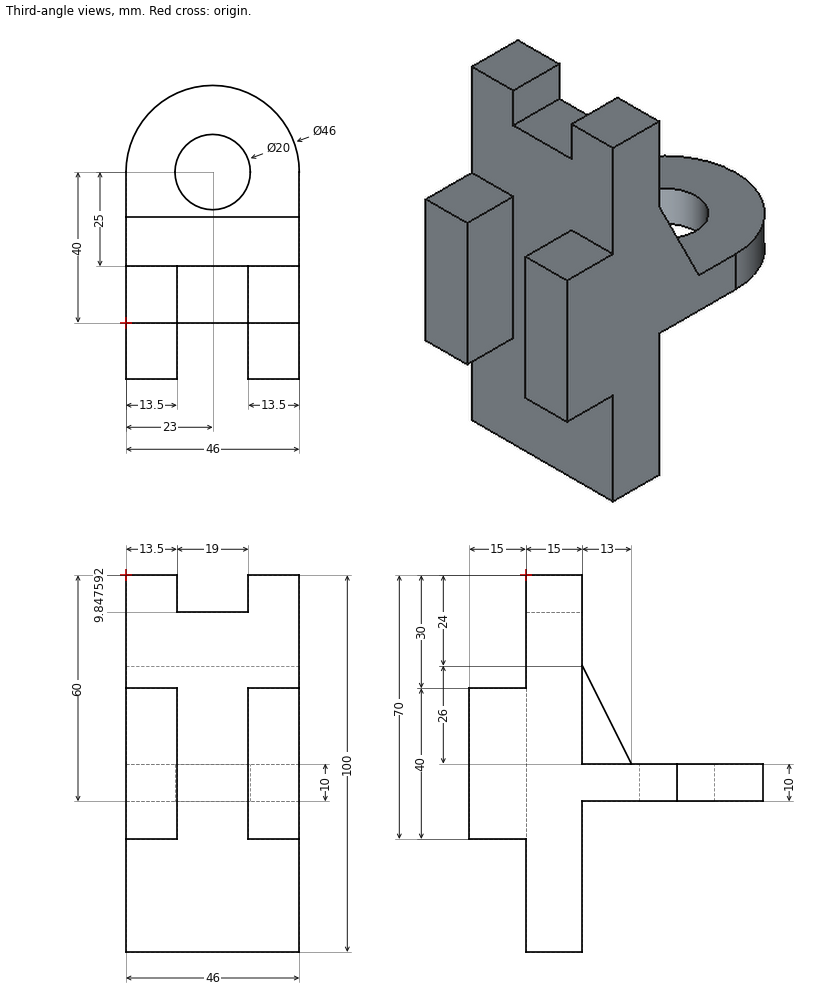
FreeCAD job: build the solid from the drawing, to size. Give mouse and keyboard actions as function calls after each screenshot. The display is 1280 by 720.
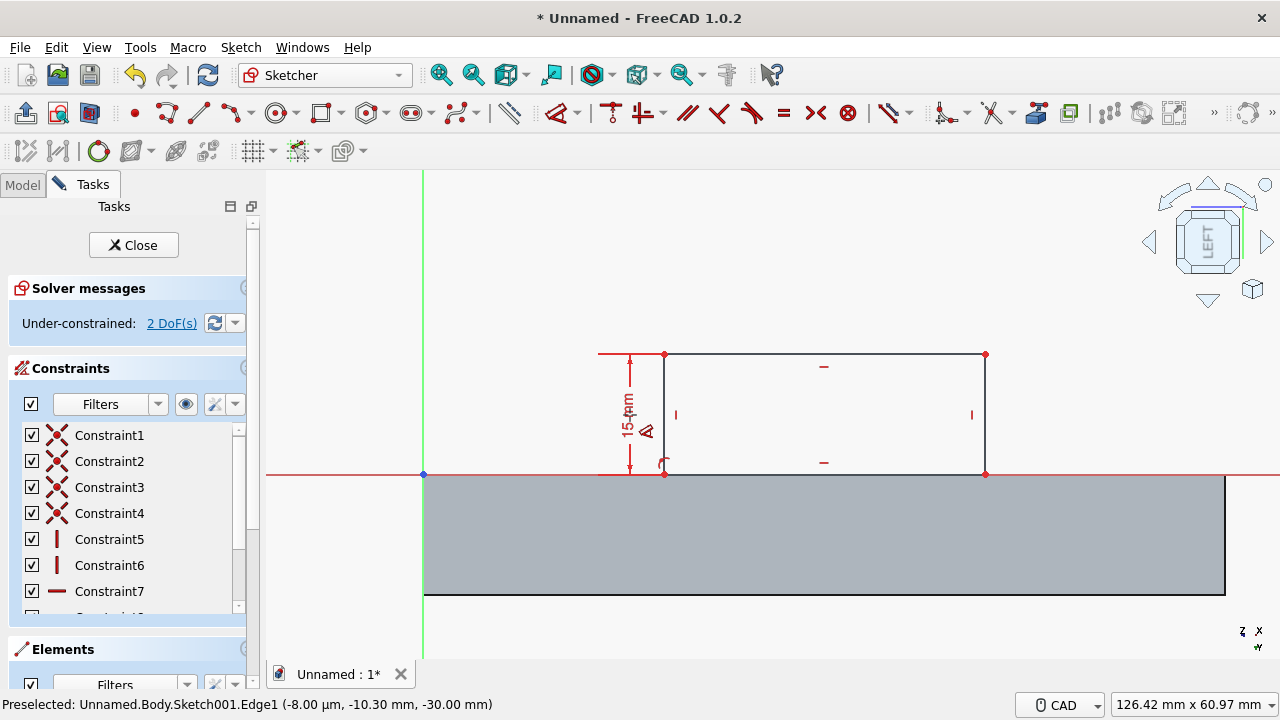
click(760, 475)
click(825, 509)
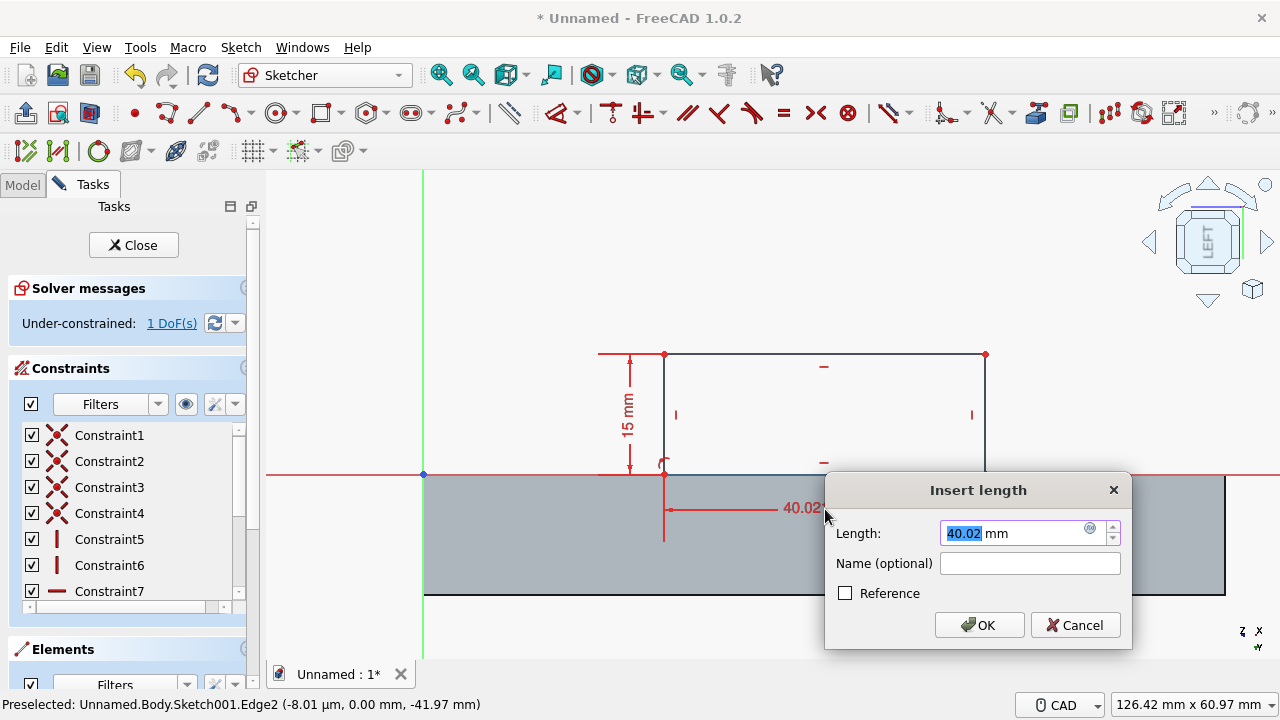
text(40)
key(Return)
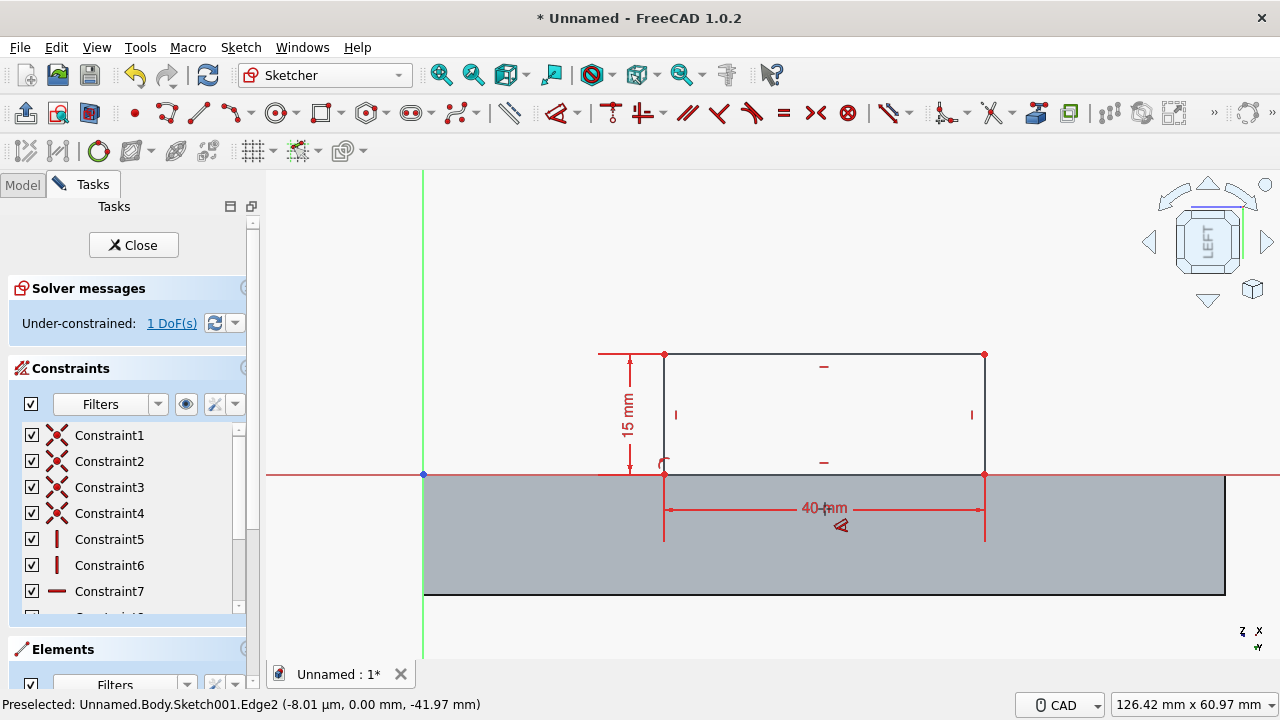
click(664, 354)
click(544, 509)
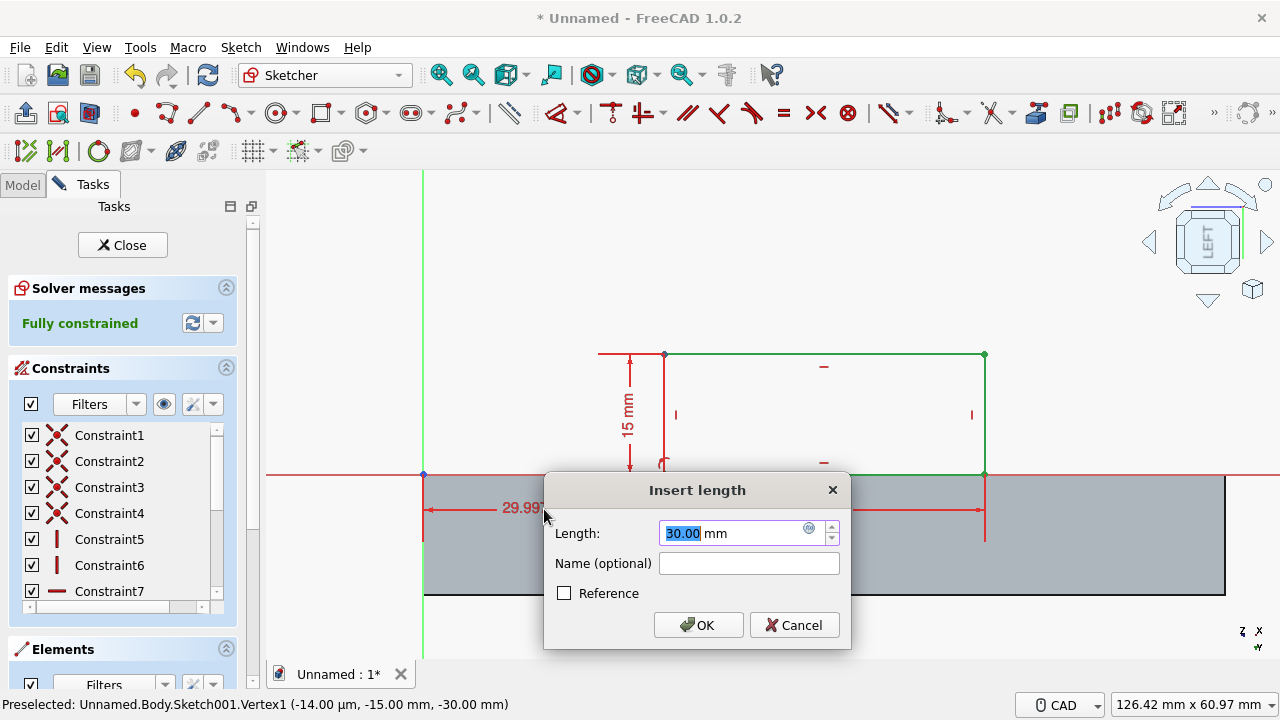
text(30)
key(Return)
key(Escape)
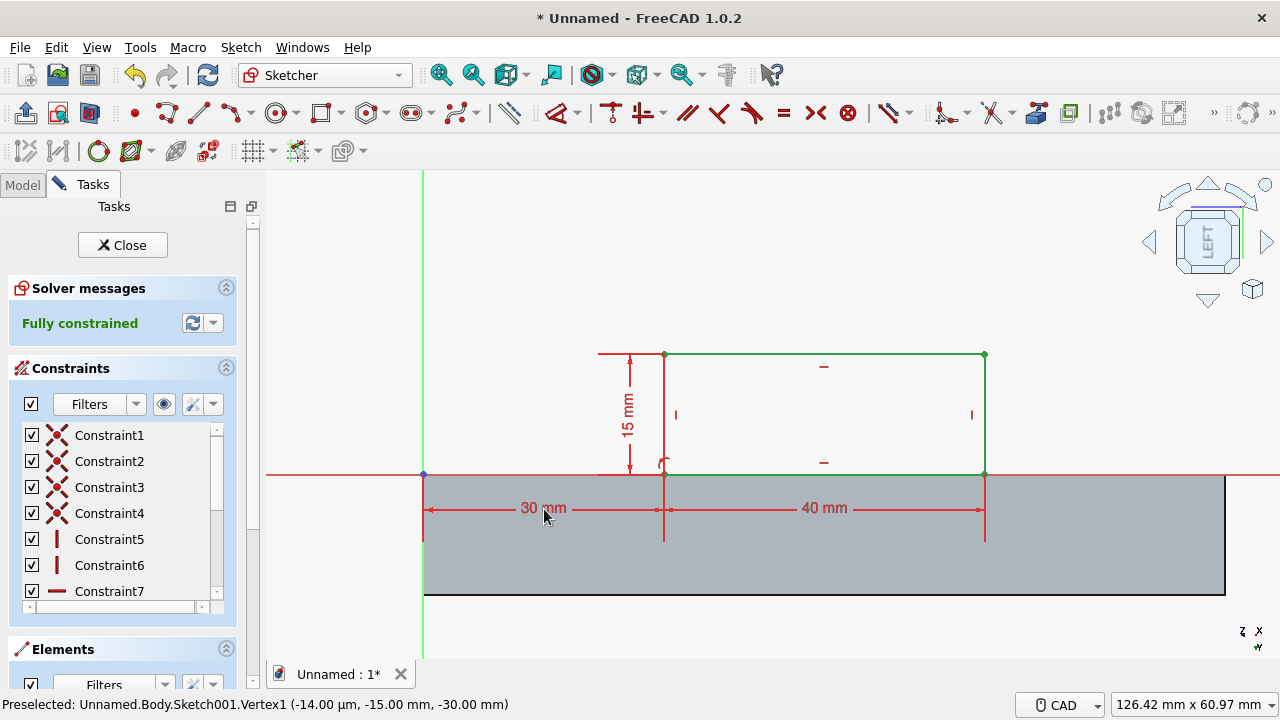
click(123, 245)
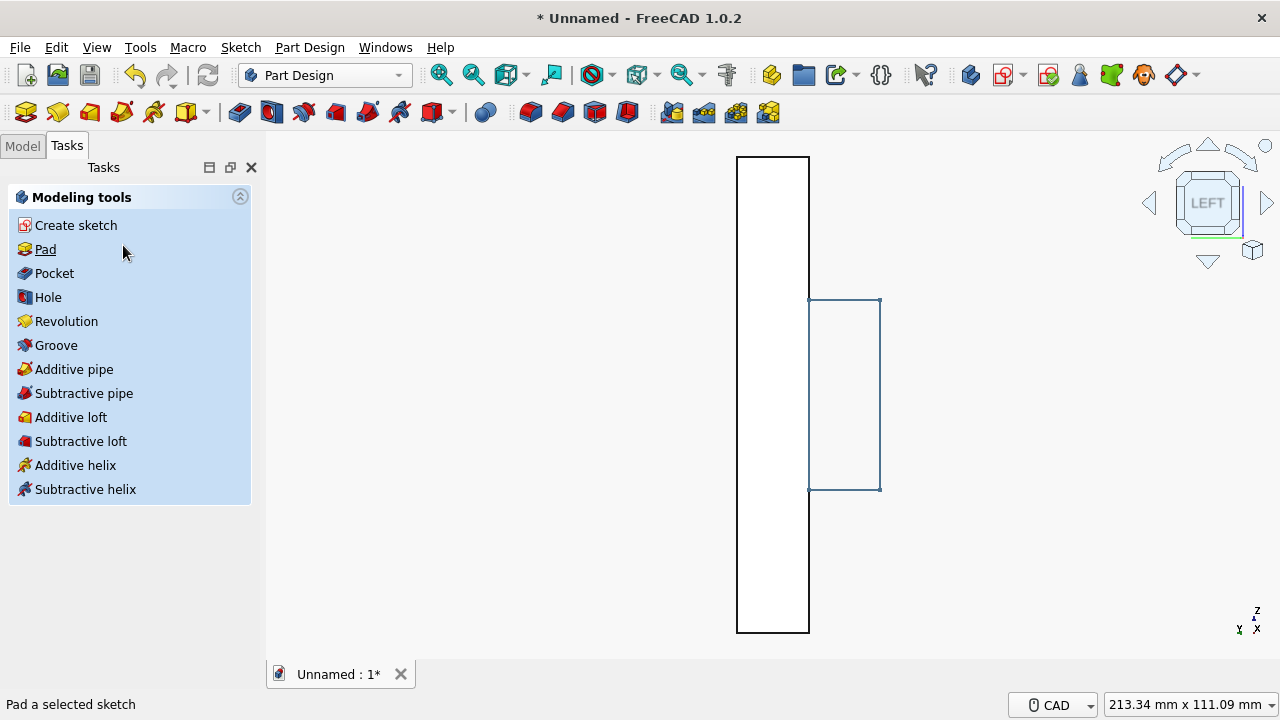
click(26, 112)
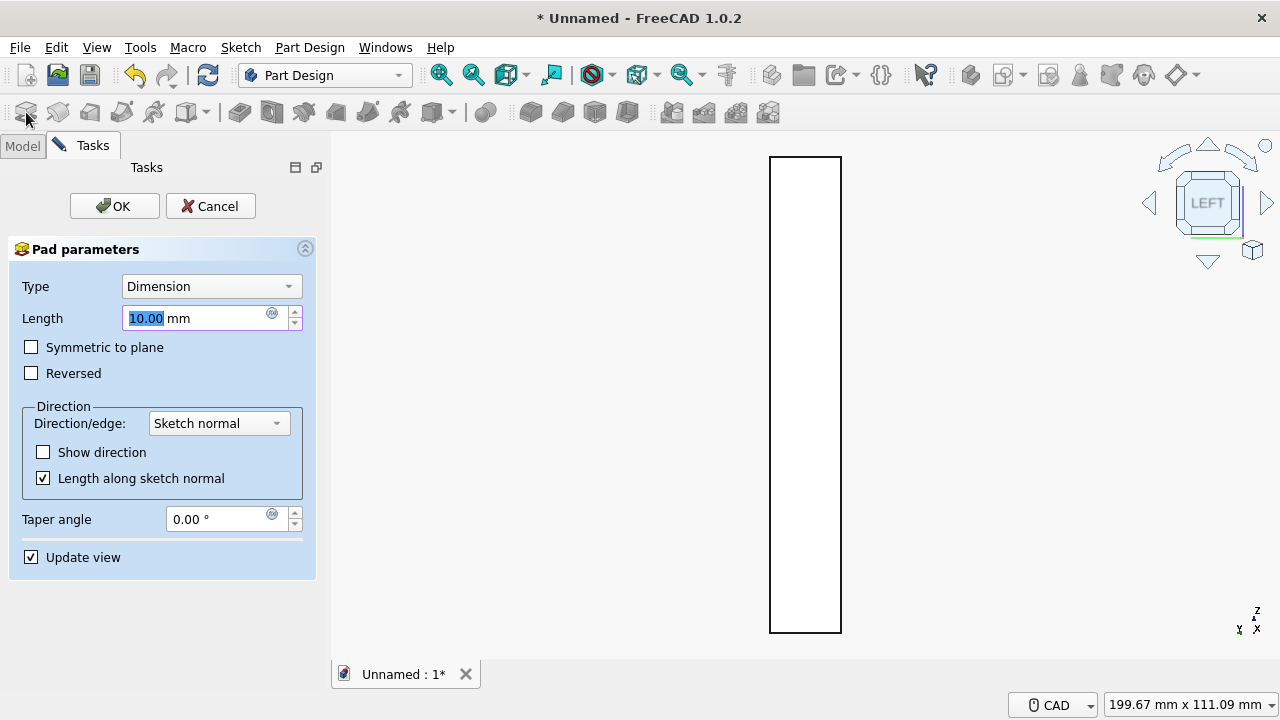
text(13.5)
key(Tab)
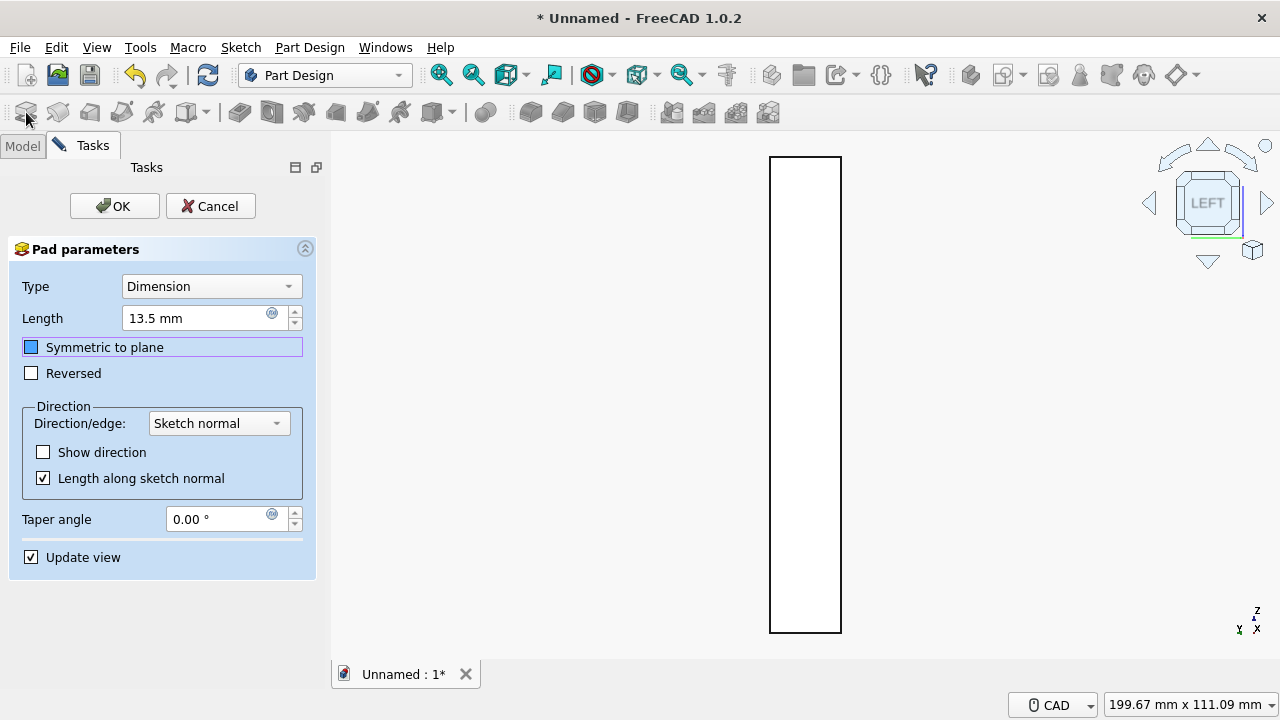
click(30, 373)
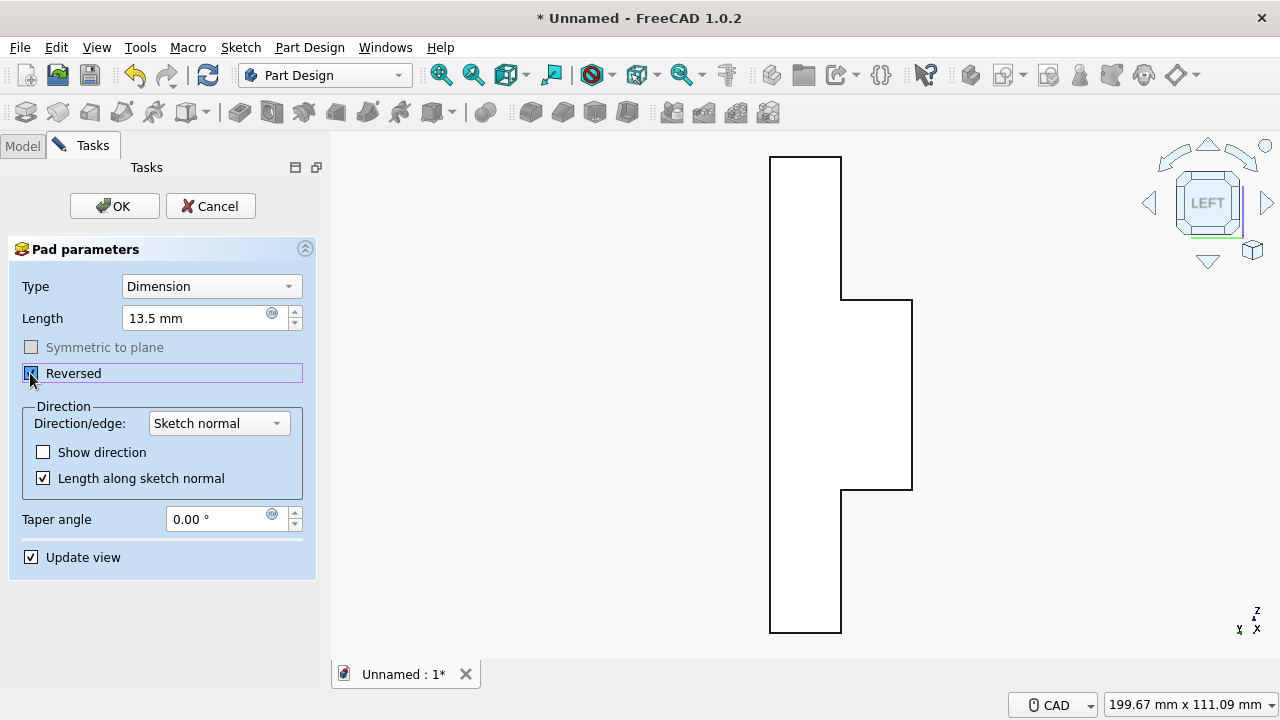
click(115, 206)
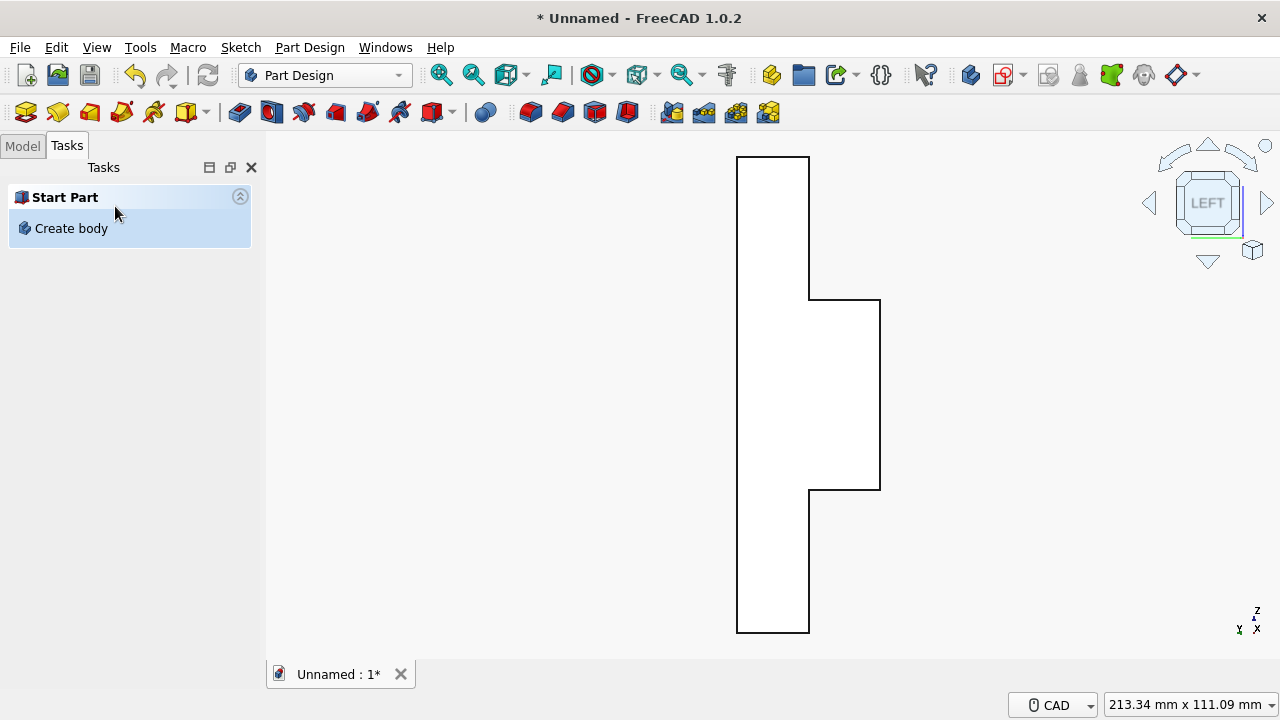
key(0)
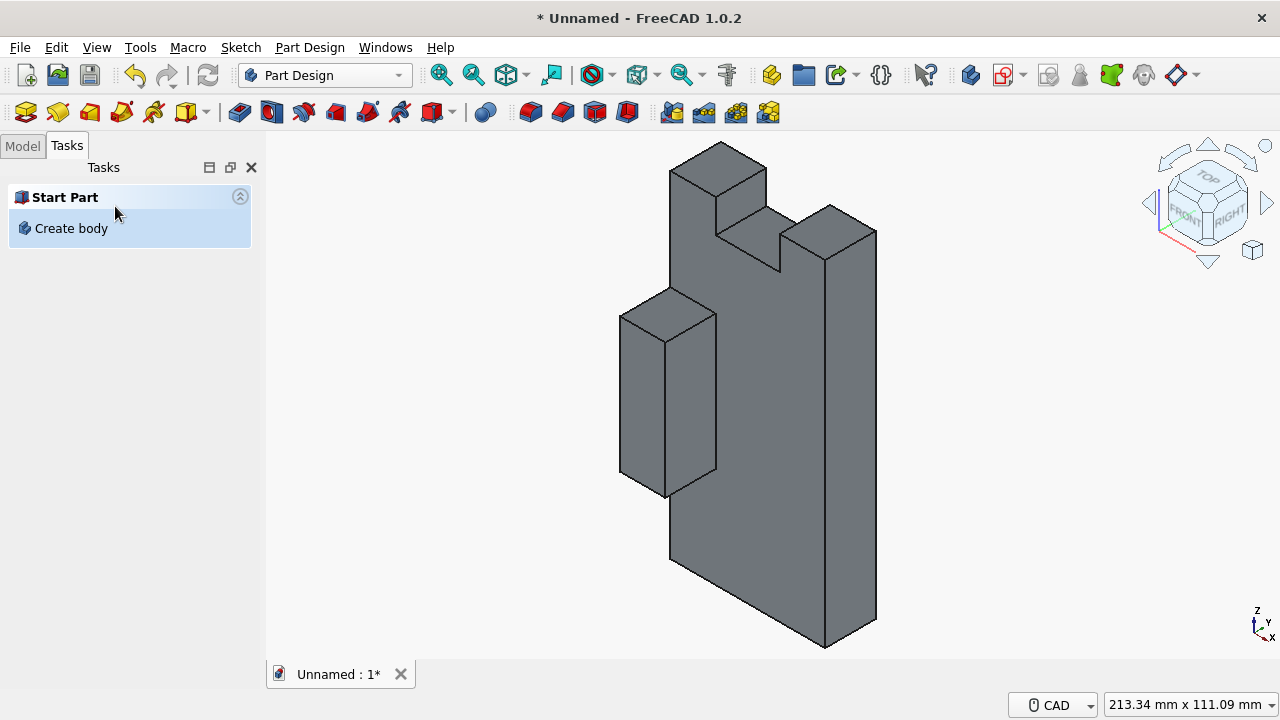
click(442, 76)